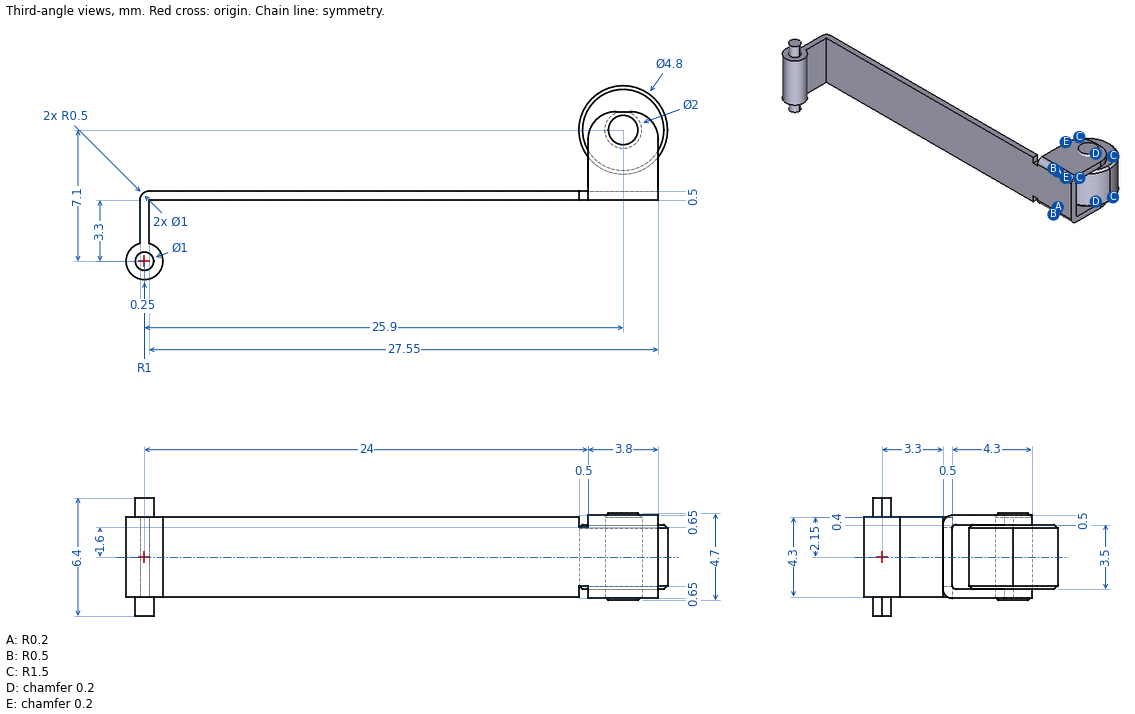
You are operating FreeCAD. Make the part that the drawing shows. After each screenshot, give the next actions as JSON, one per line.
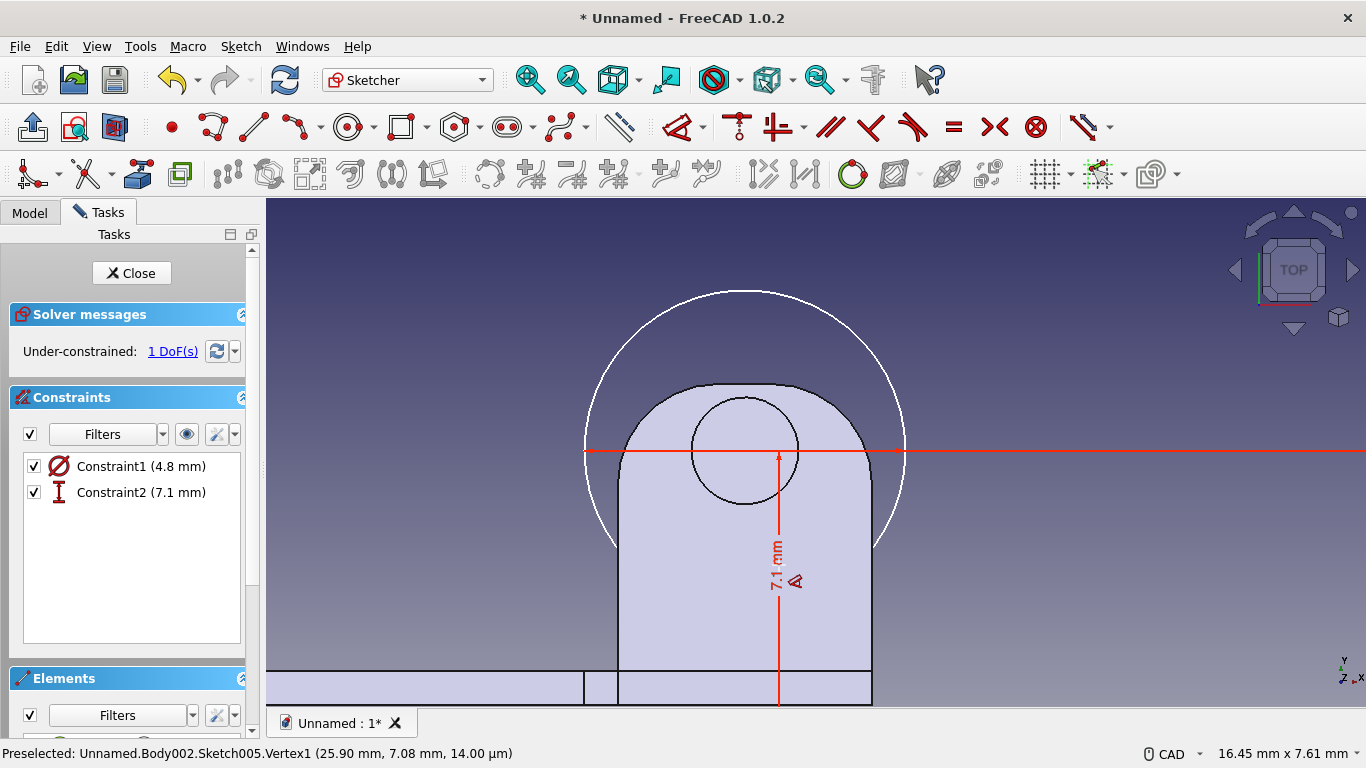
{"action": "left_click", "coordinate": [745, 451]}
{"action": "left_click", "coordinate": [520, 417]}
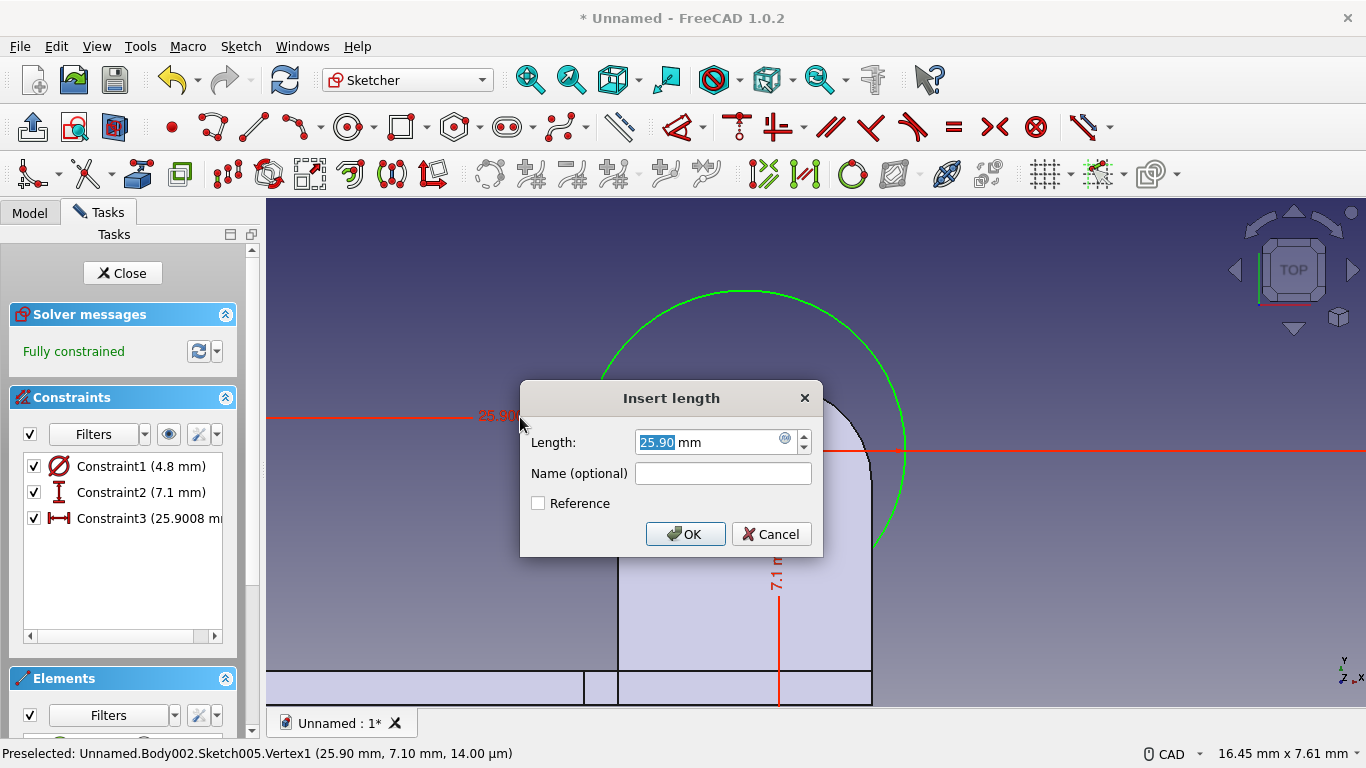
{"action": "type", "text": "25.9"}
{"action": "key", "text": "Return"}
{"action": "key", "text": "Escape"}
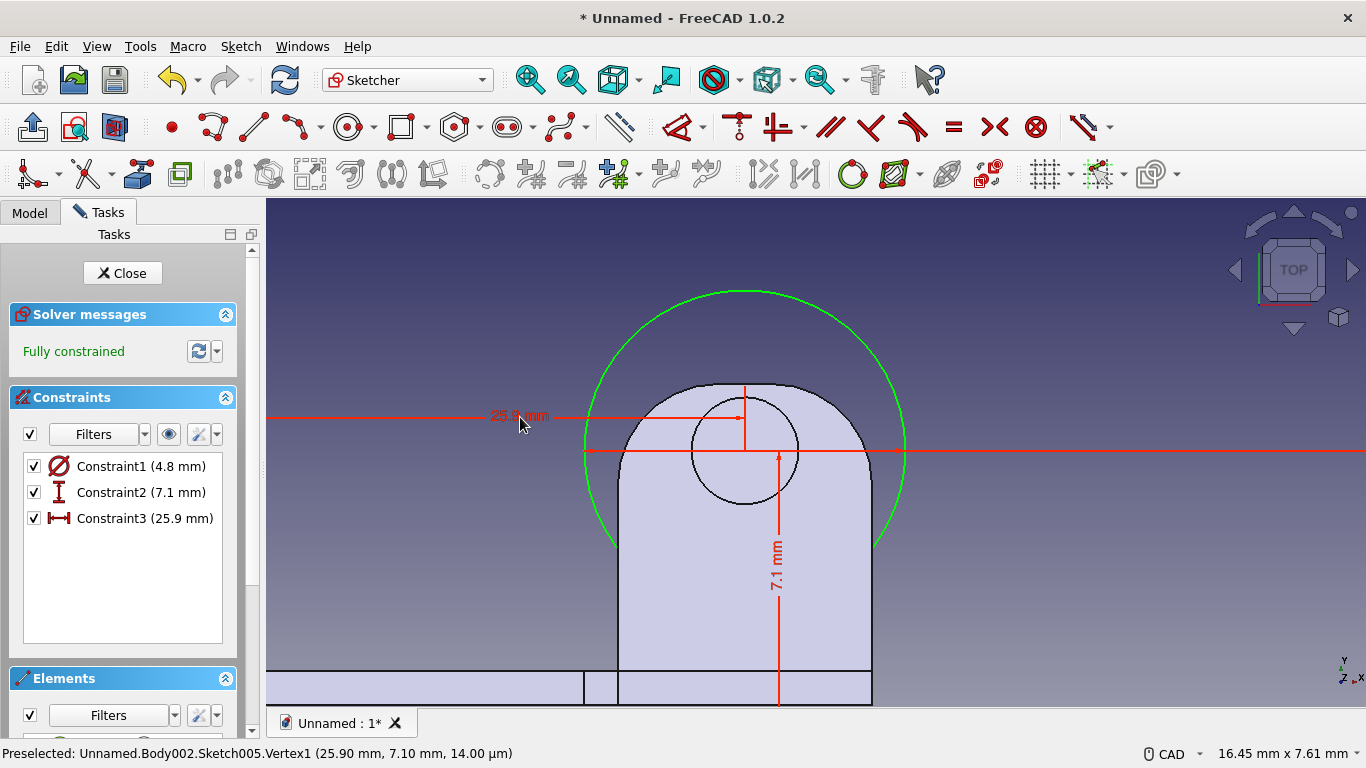
{"action": "left_click", "coordinate": [123, 273]}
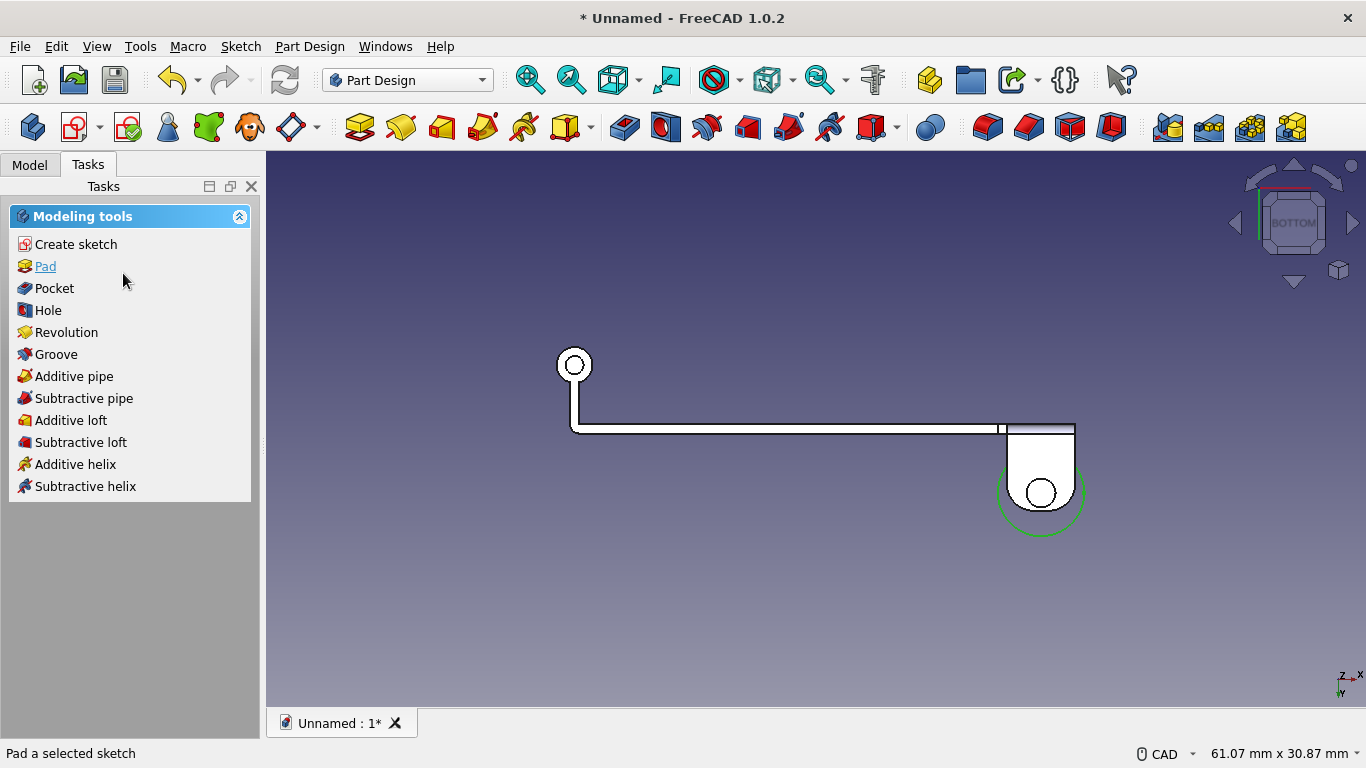
{"action": "left_click", "coordinate": [360, 128]}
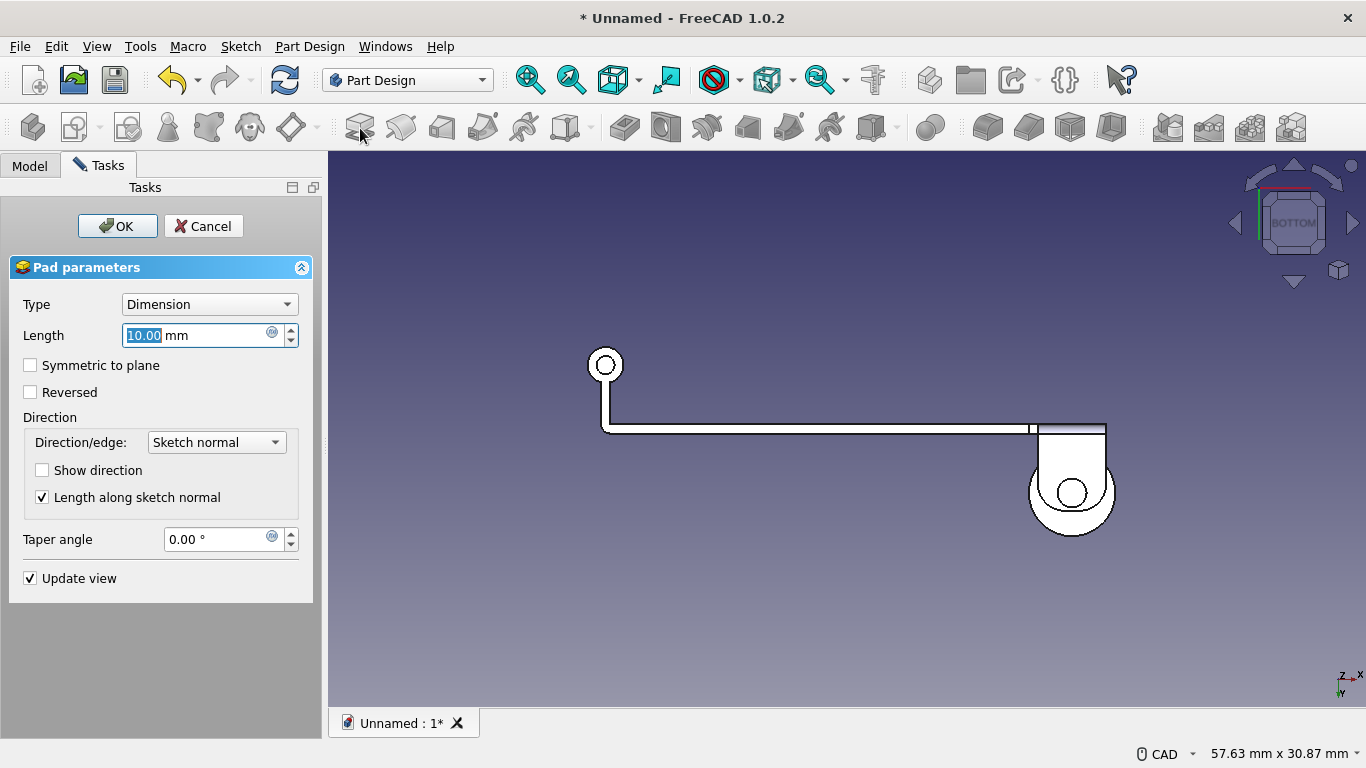
{"action": "type", "text": "3.5"}
{"action": "key", "text": "Tab"}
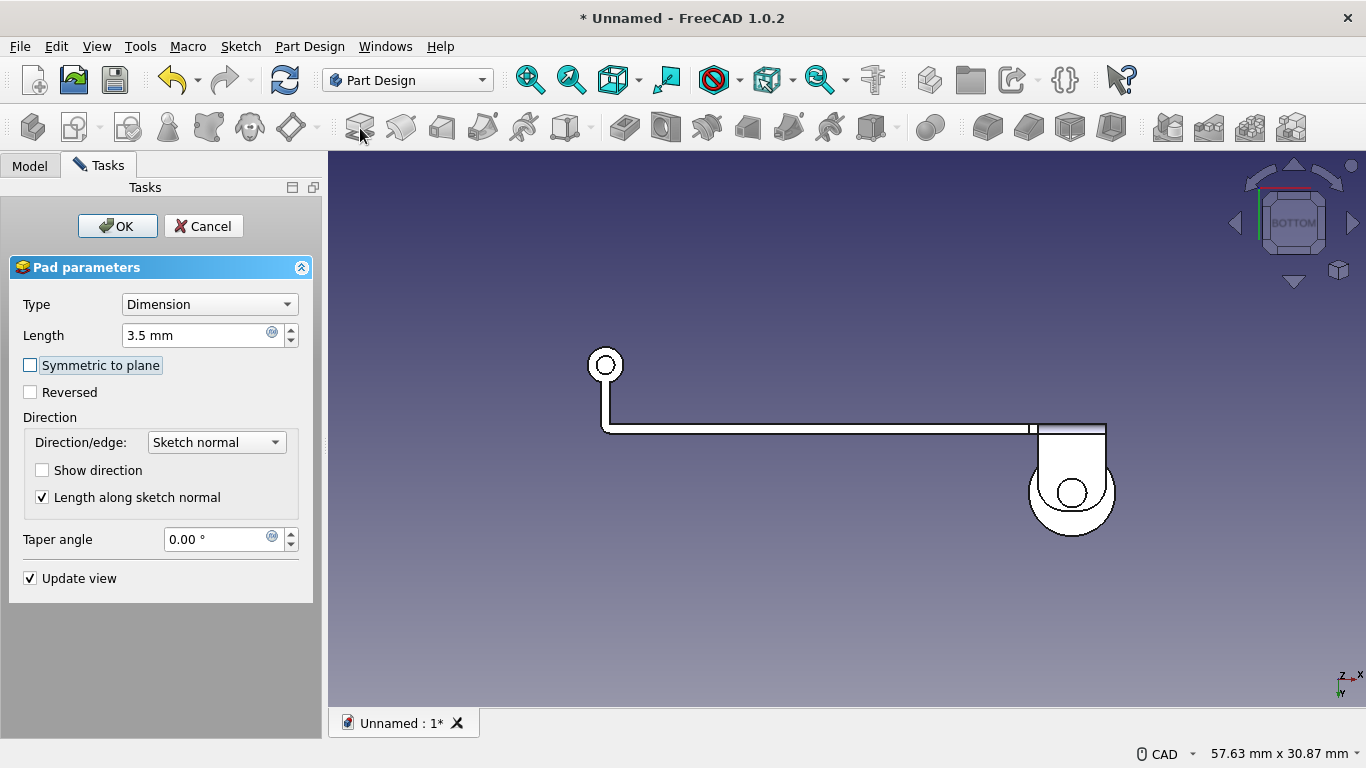
{"action": "left_click", "coordinate": [31, 365]}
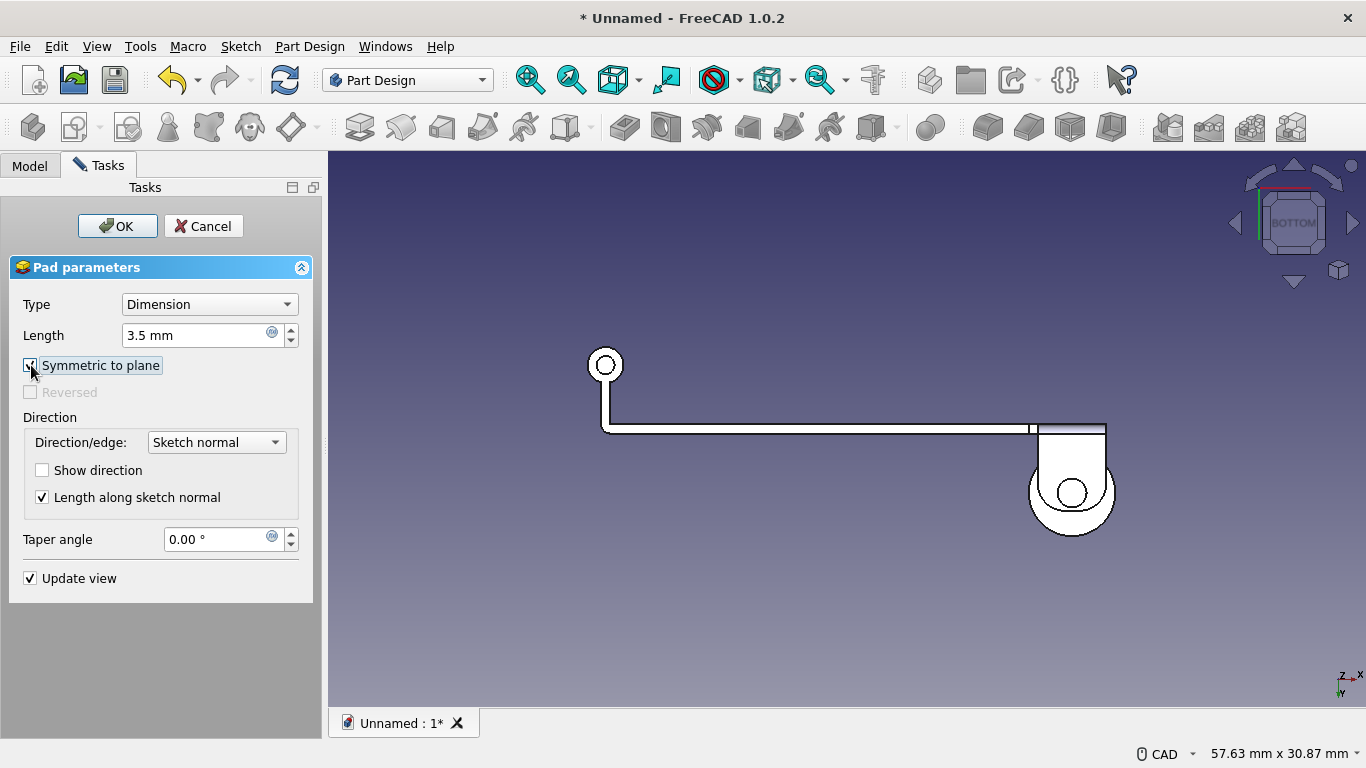
{"action": "left_click", "coordinate": [118, 226]}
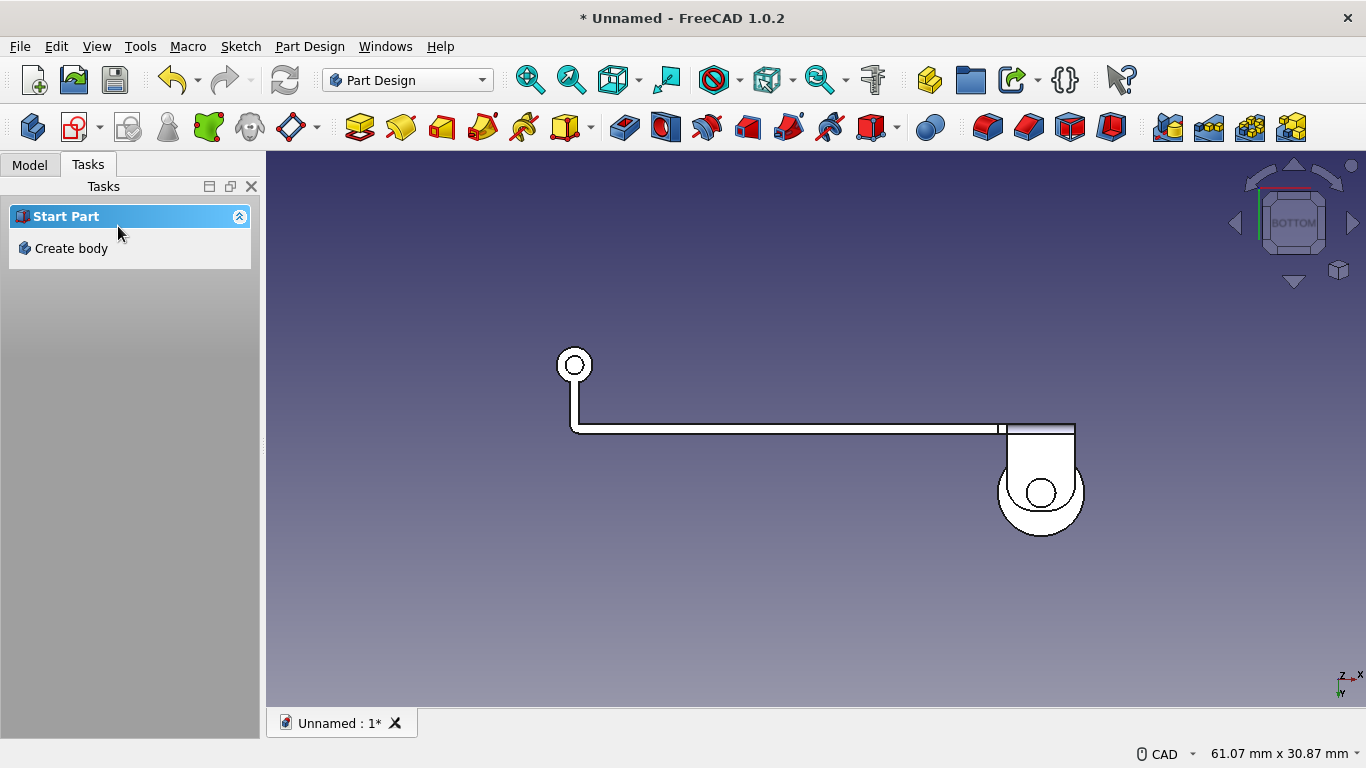
{"action": "left_click", "coordinate": [531, 80]}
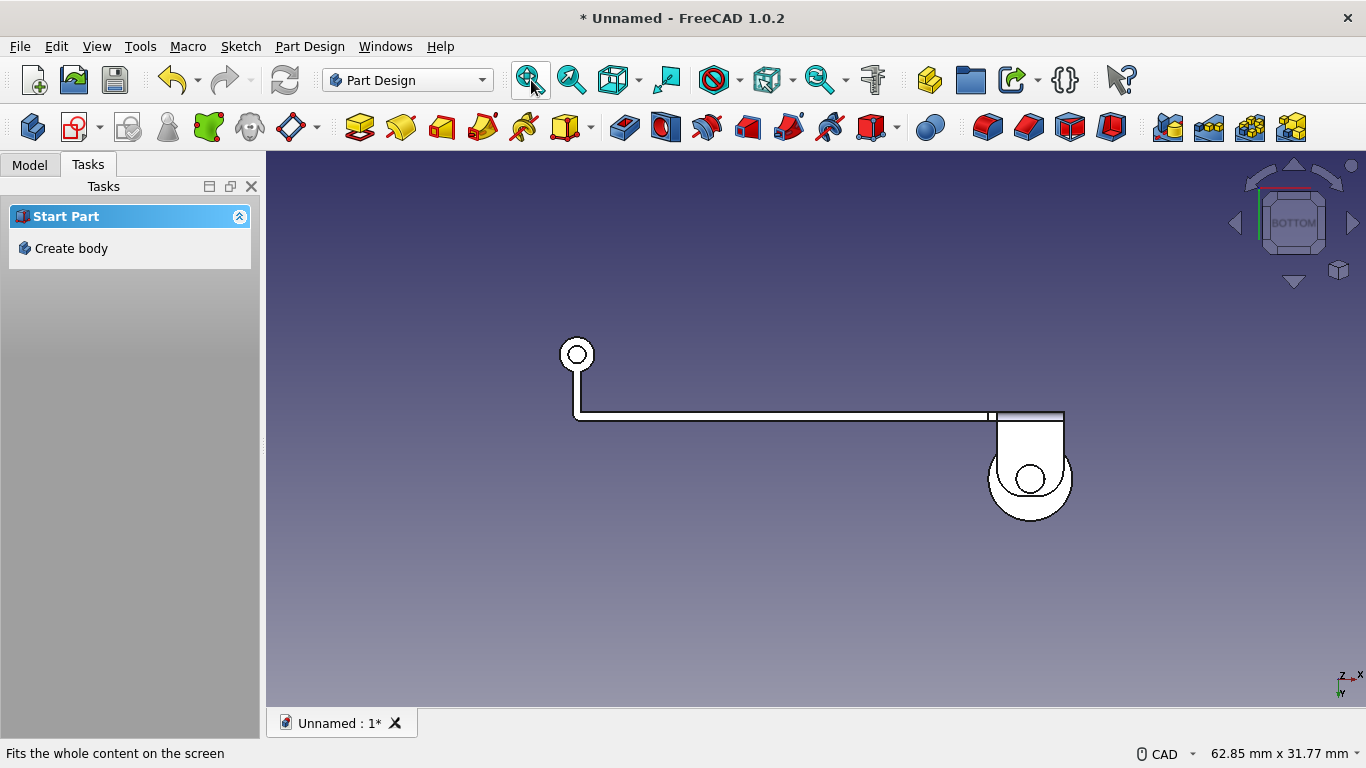
{"action": "left_click", "coordinate": [988, 478]}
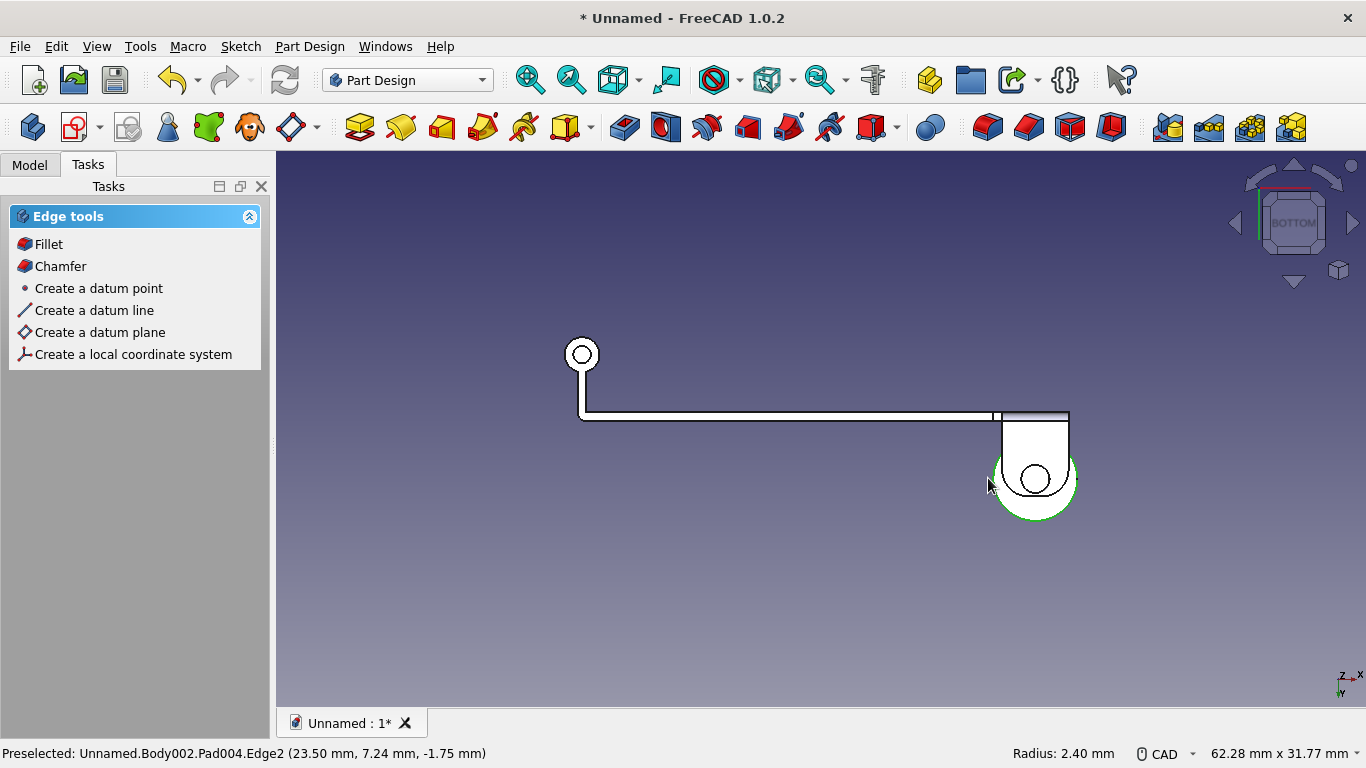
{"action": "key", "text": "0"}